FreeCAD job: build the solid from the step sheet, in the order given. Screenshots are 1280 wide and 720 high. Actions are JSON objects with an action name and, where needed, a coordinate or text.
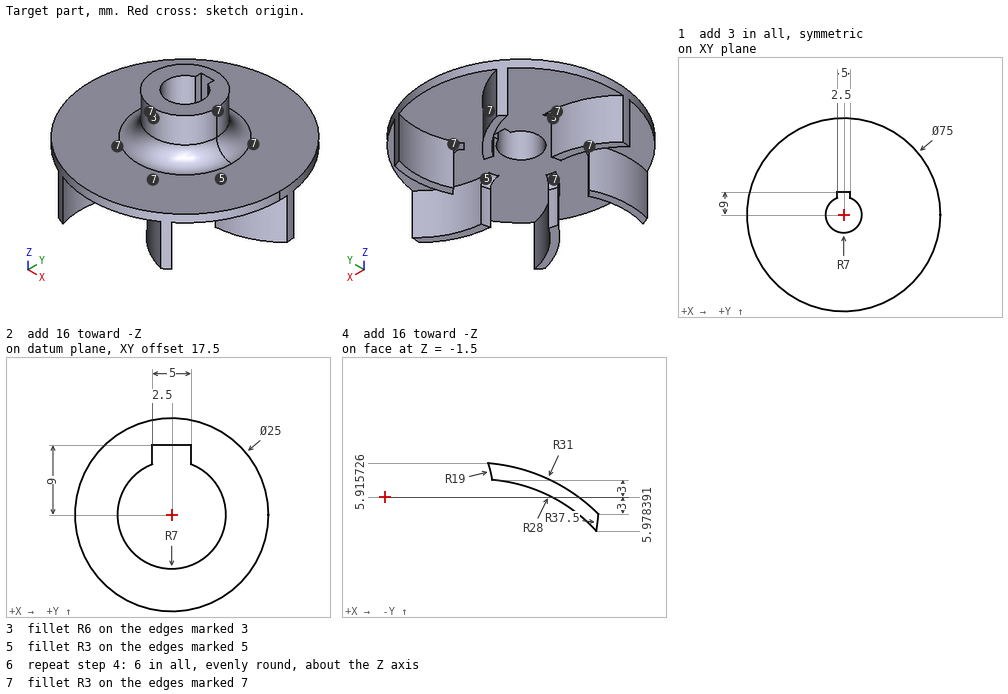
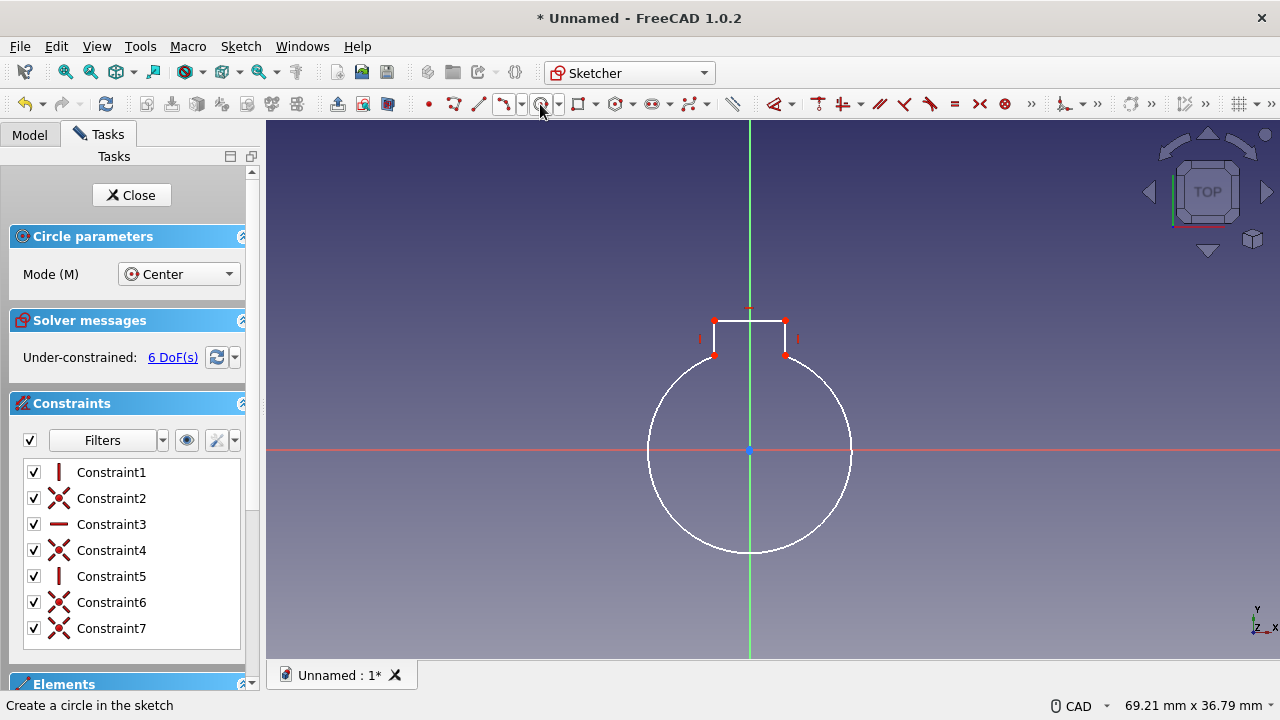
{"action": "left_click", "coordinate": [750, 450]}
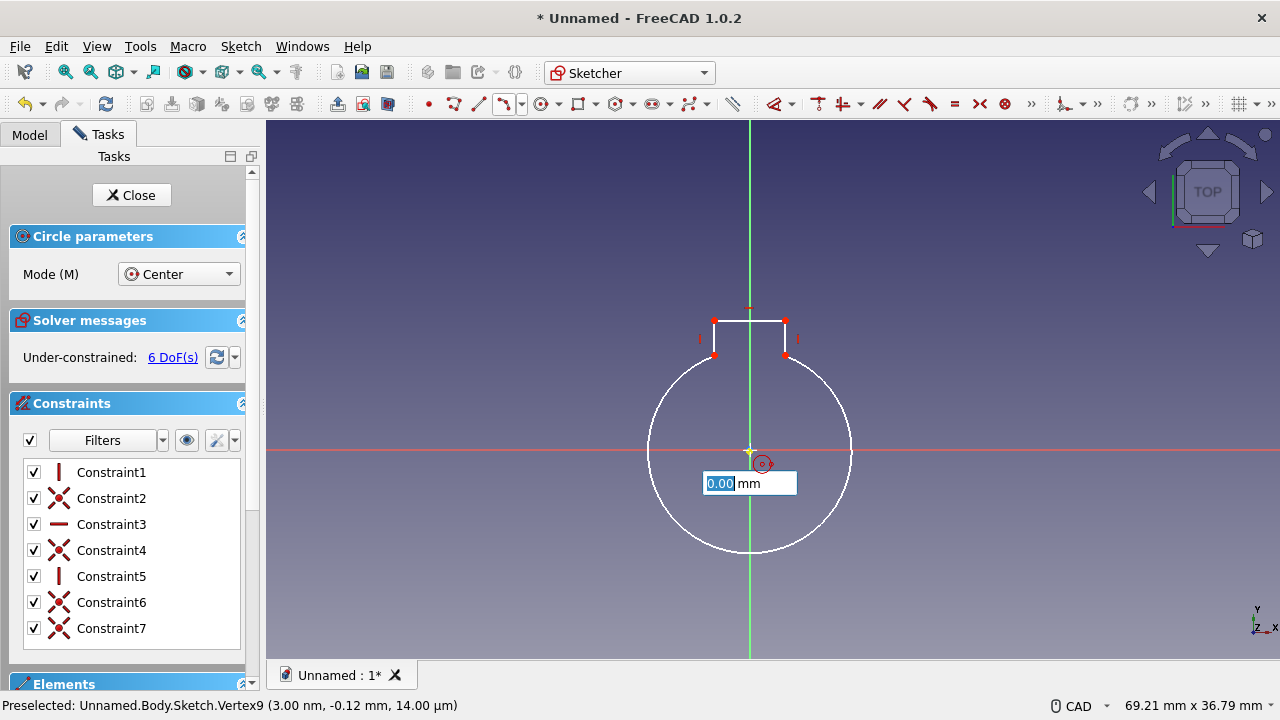
{"action": "scroll", "coordinate": [685, 364], "scroll_direction": "down", "scroll_amount": 6}
{"action": "mouse_move", "coordinate": [822, 273]}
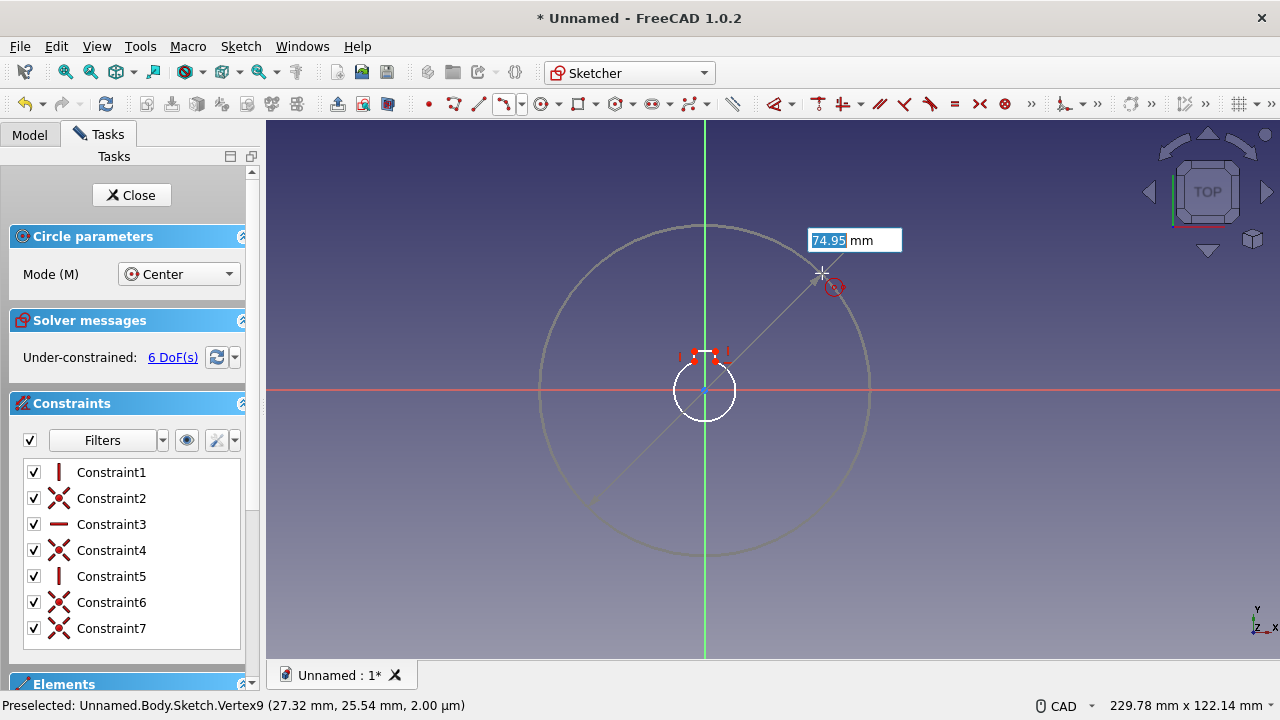
{"action": "type", "text": "75"}
{"action": "key", "text": "Return"}
{"action": "key", "text": "Escape"}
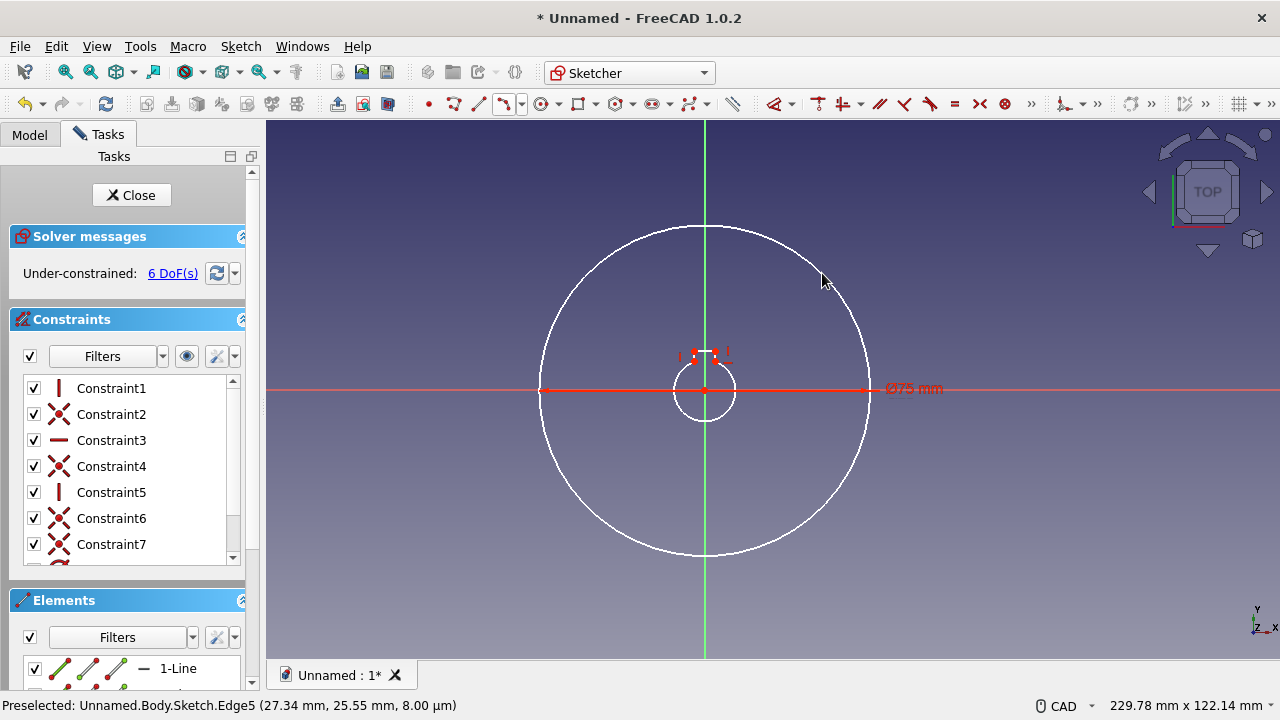
{"action": "scroll", "coordinate": [705, 390], "scroll_direction": "up", "scroll_amount": 2}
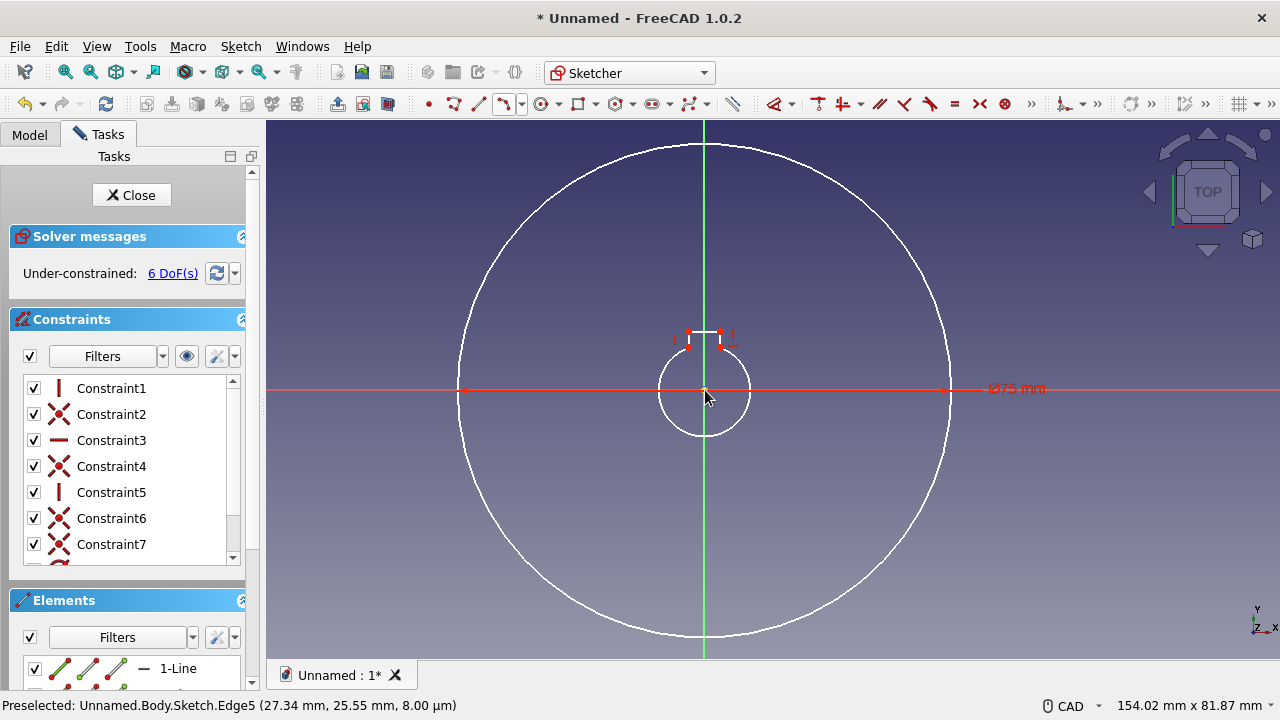
{"action": "left_click_drag", "start_coordinate": [694, 380], "coordinate": [714, 401]}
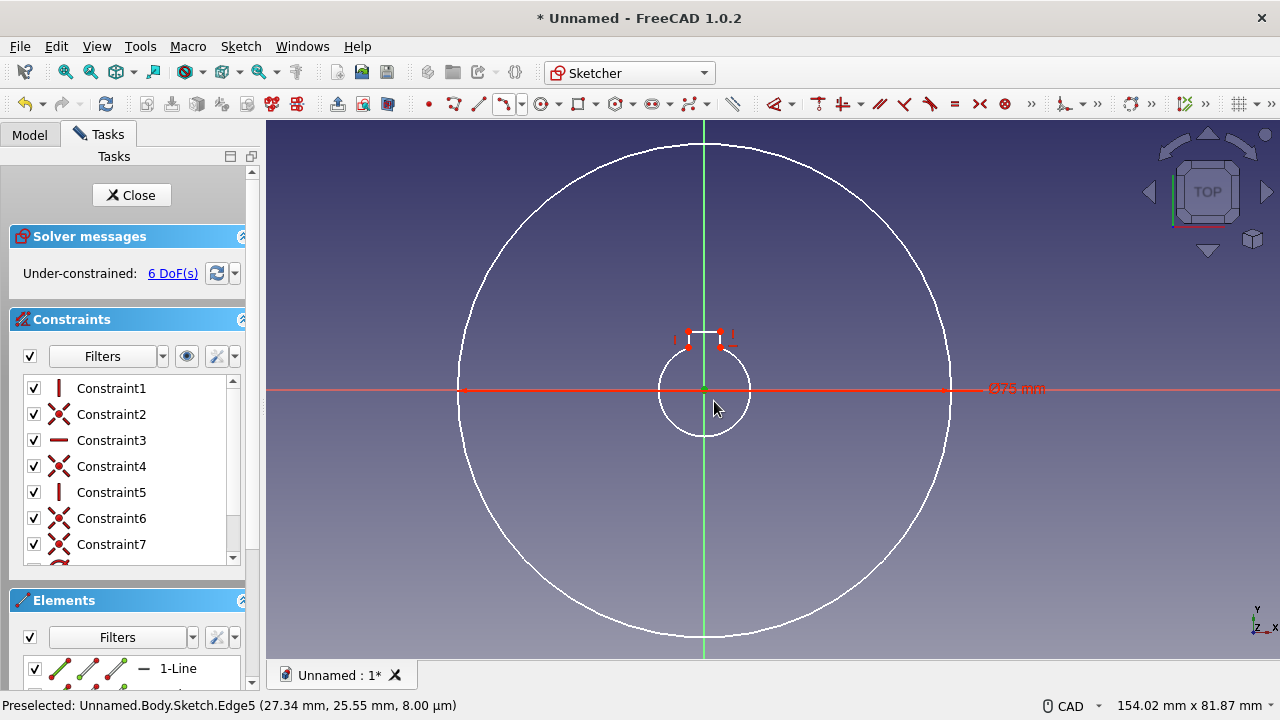
{"action": "left_click", "coordinate": [818, 104]}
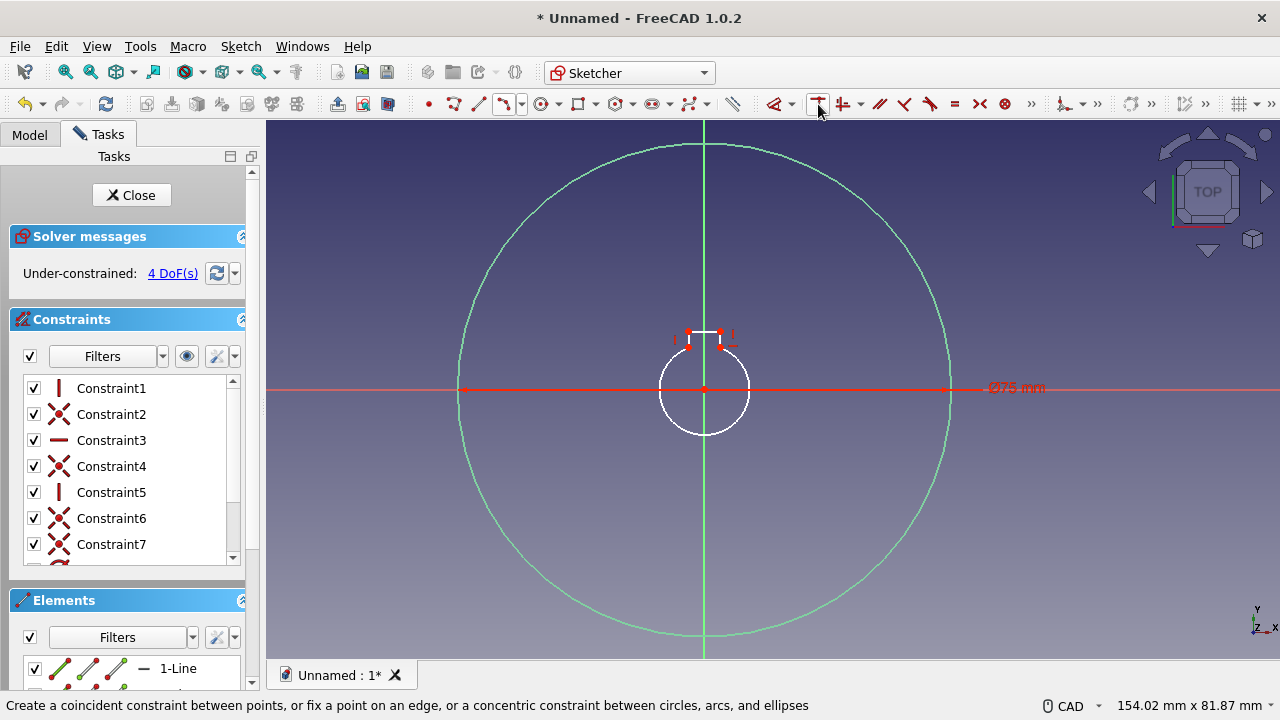
{"action": "left_click", "coordinate": [774, 104]}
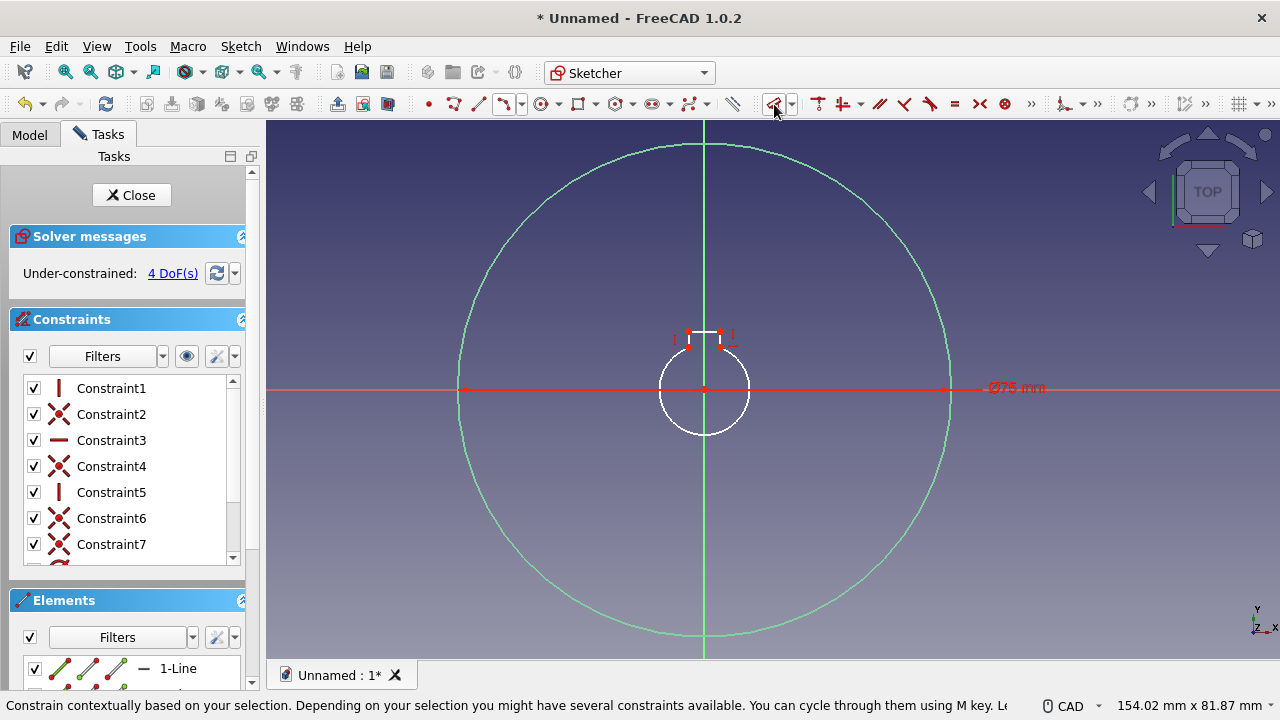
{"action": "left_click", "coordinate": [664, 410]}
{"action": "left_click", "coordinate": [635, 424]}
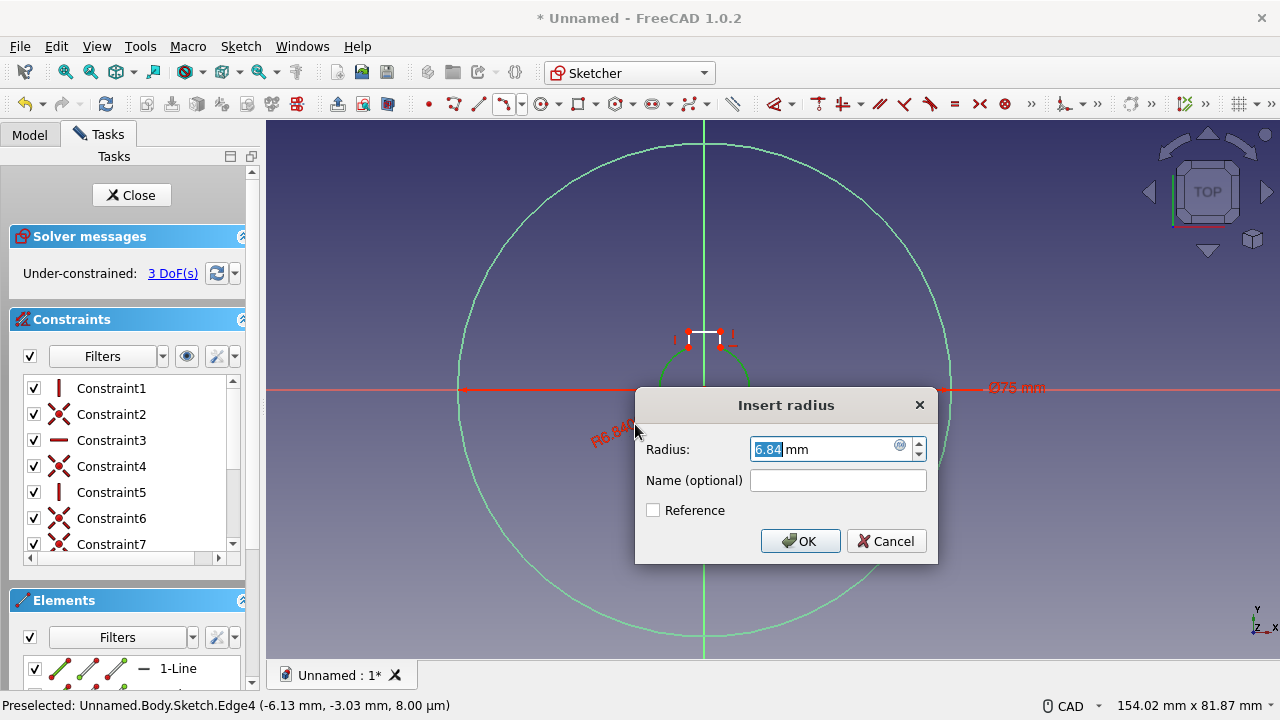
{"action": "type", "text": "7"}
{"action": "key", "text": "Return"}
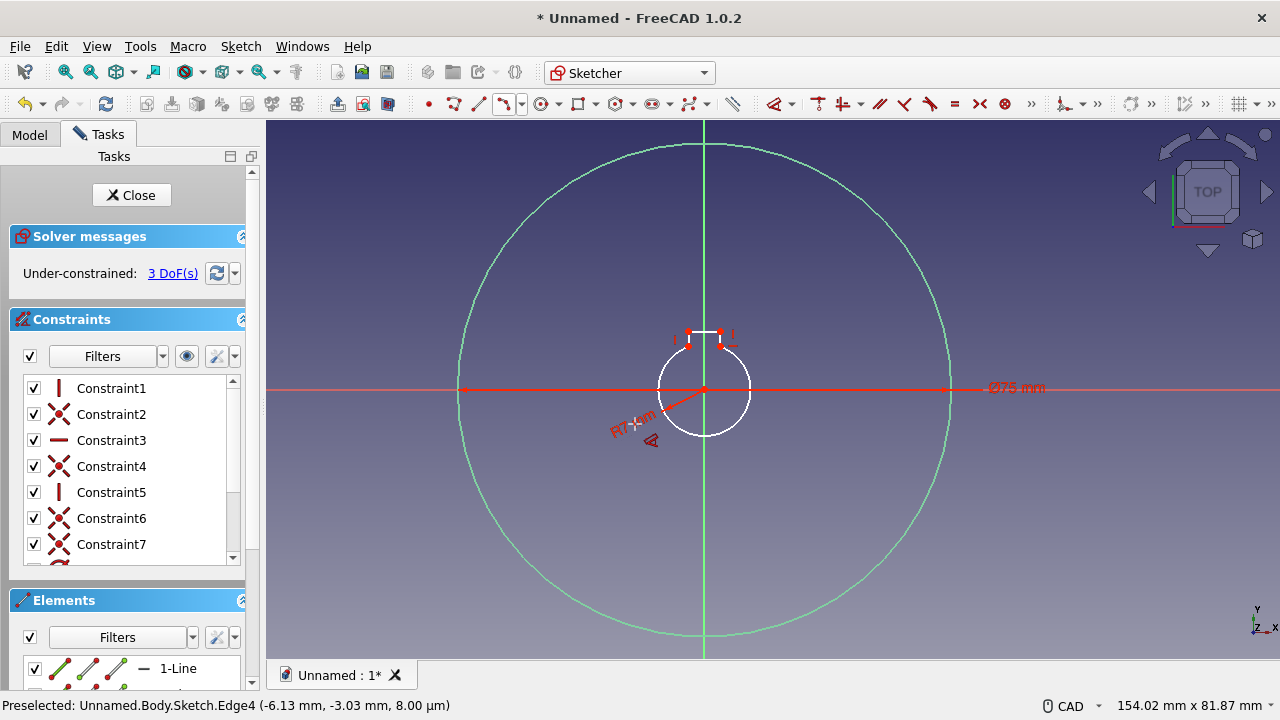
{"action": "left_click", "coordinate": [701, 332]}
{"action": "left_click", "coordinate": [697, 298]}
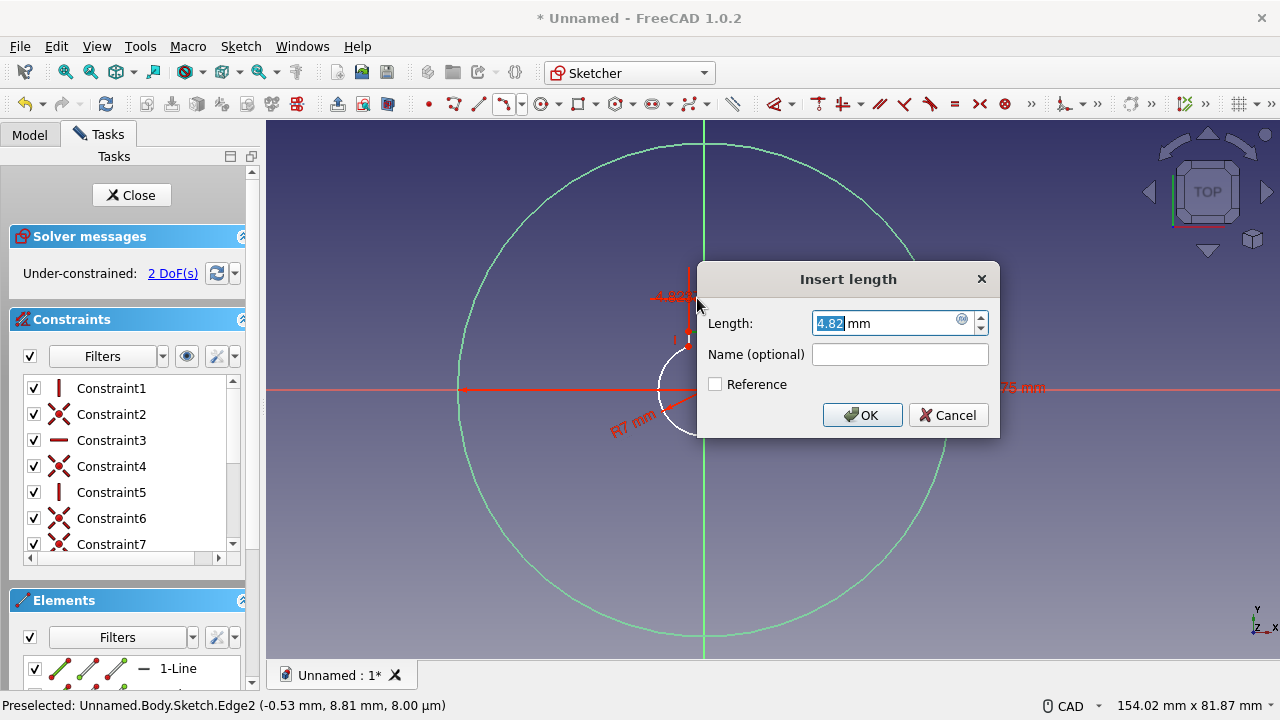
{"action": "type", "text": "5"}
{"action": "key", "text": "Return"}